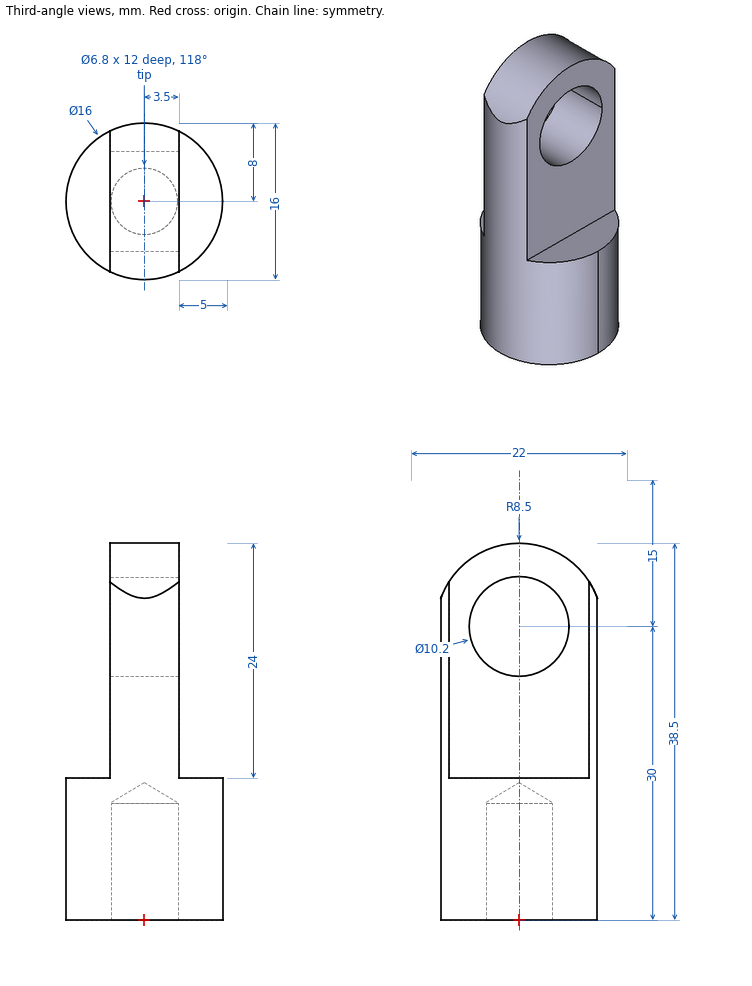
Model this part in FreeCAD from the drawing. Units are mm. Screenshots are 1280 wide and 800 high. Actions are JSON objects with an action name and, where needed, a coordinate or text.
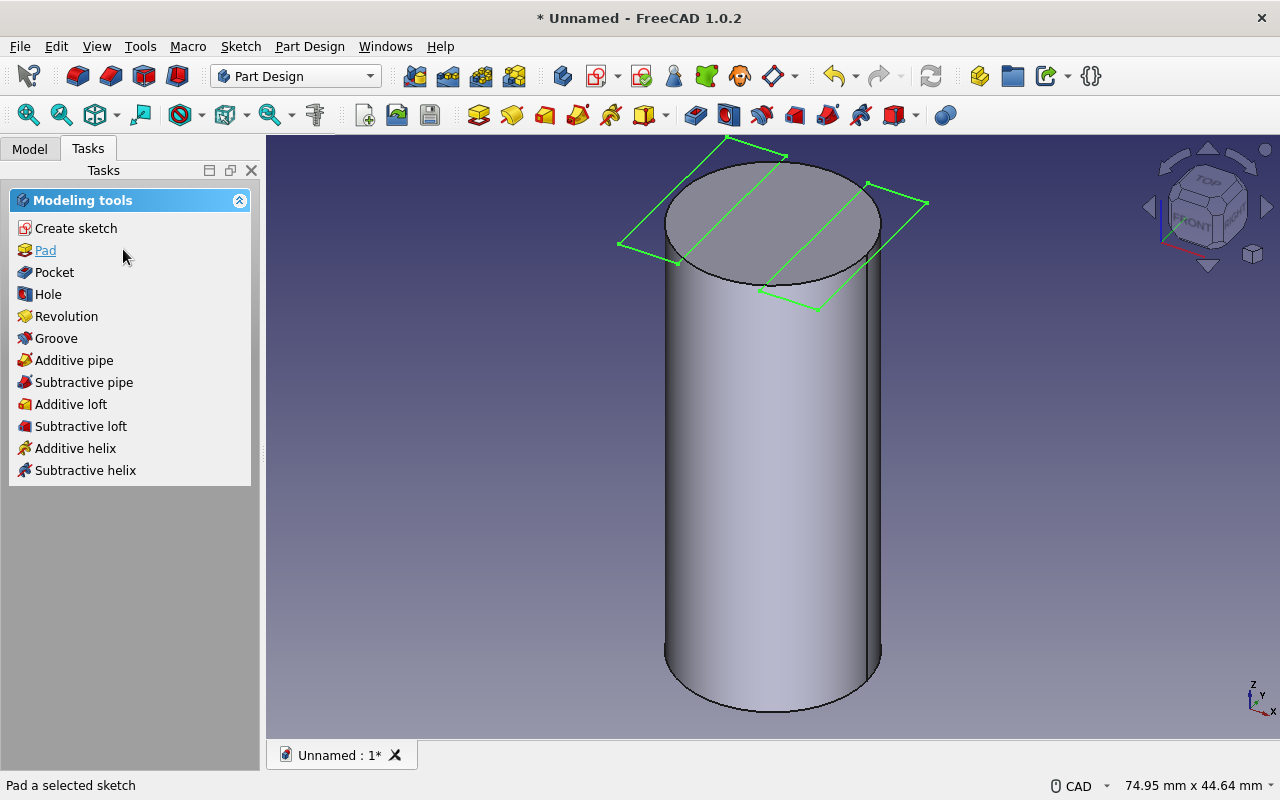
{"action": "left_click", "coordinate": [696, 116]}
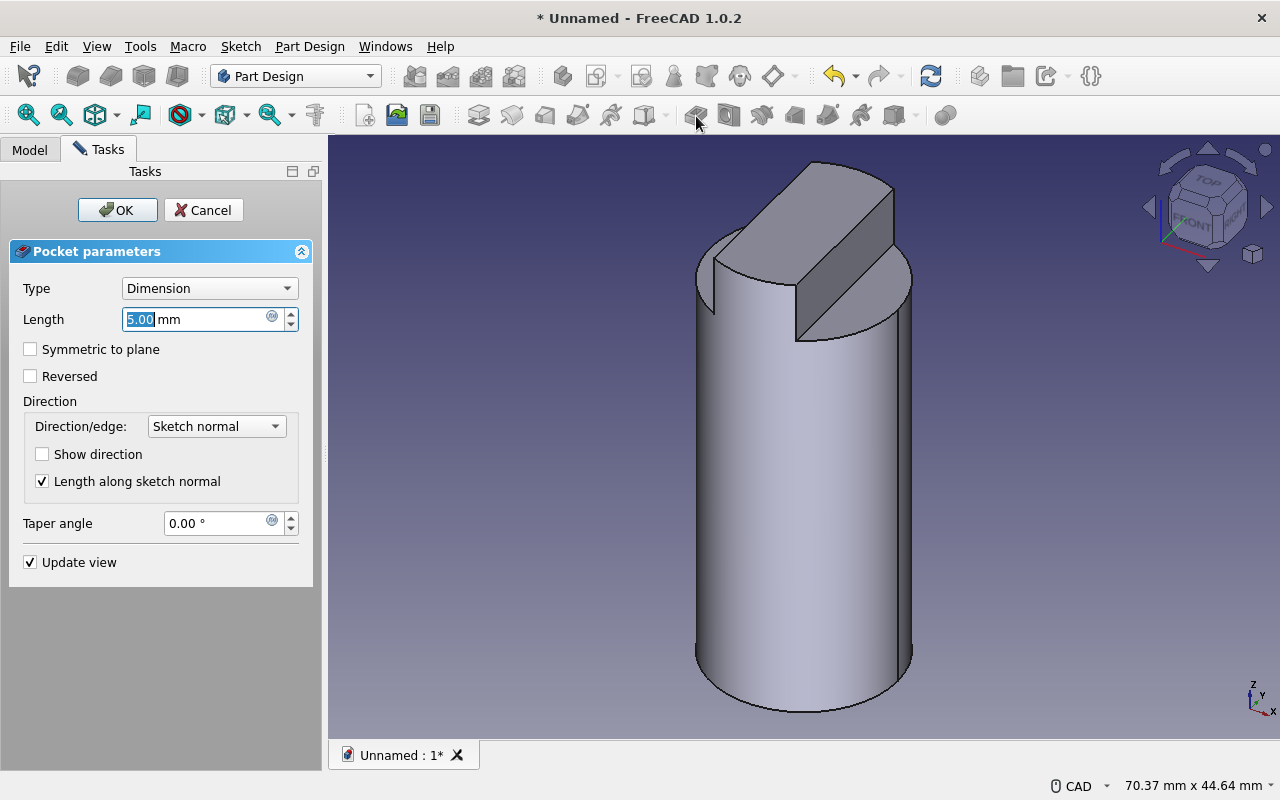
{"action": "type", "text": "24"}
{"action": "key", "text": "Tab"}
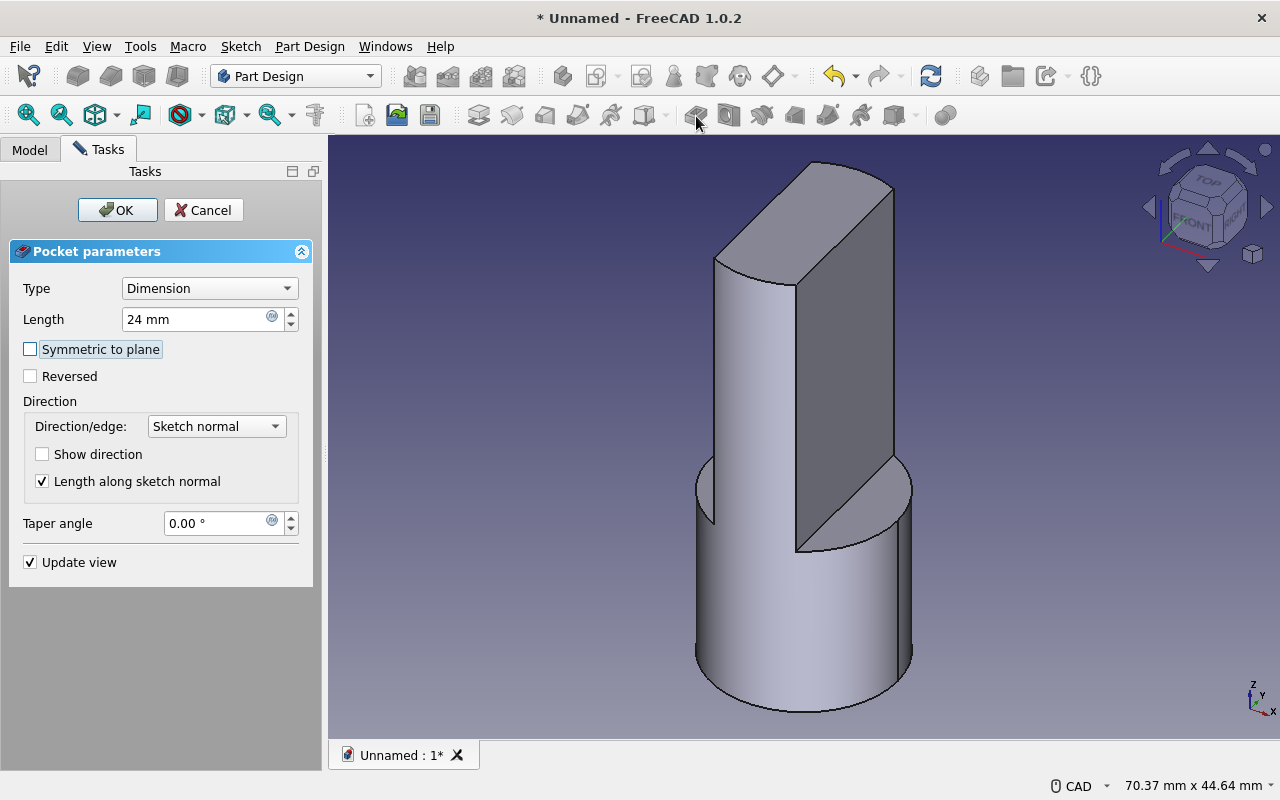
{"action": "left_click", "coordinate": [118, 210]}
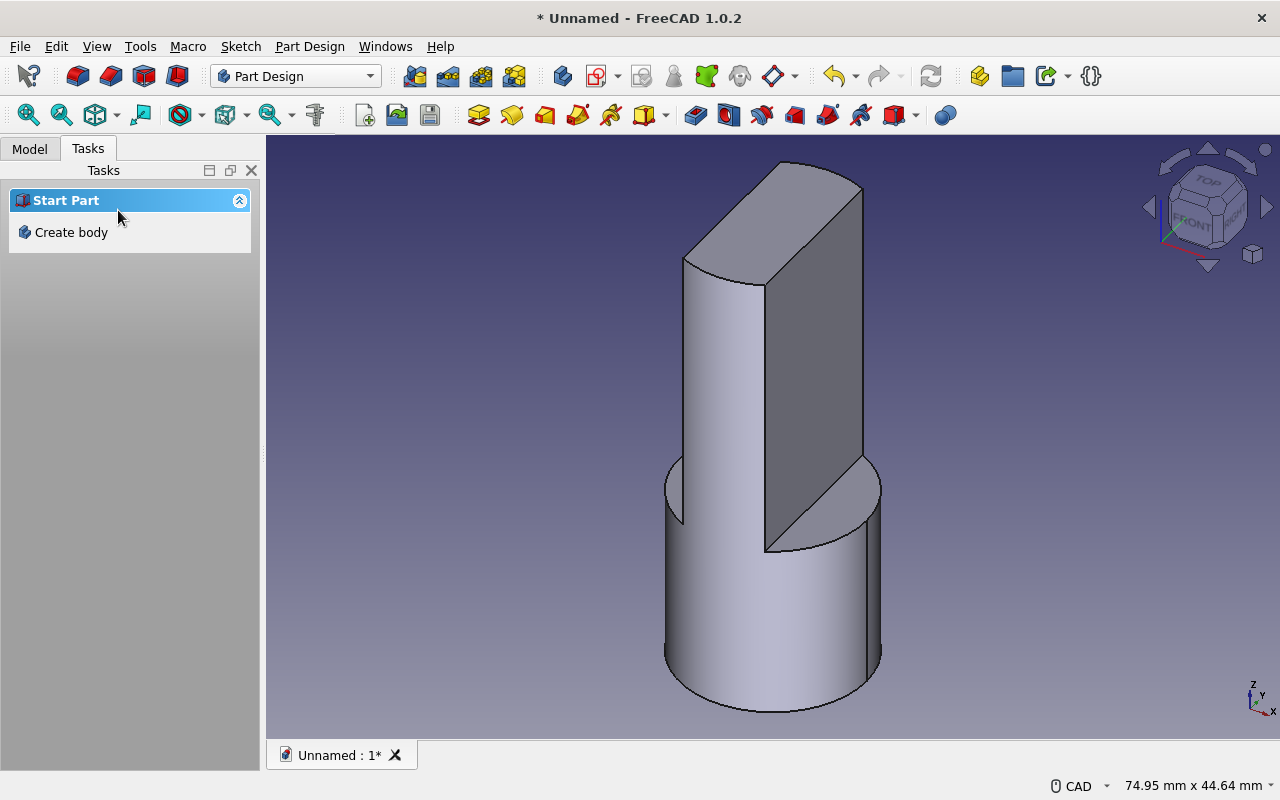
{"action": "left_click", "coordinate": [814, 331]}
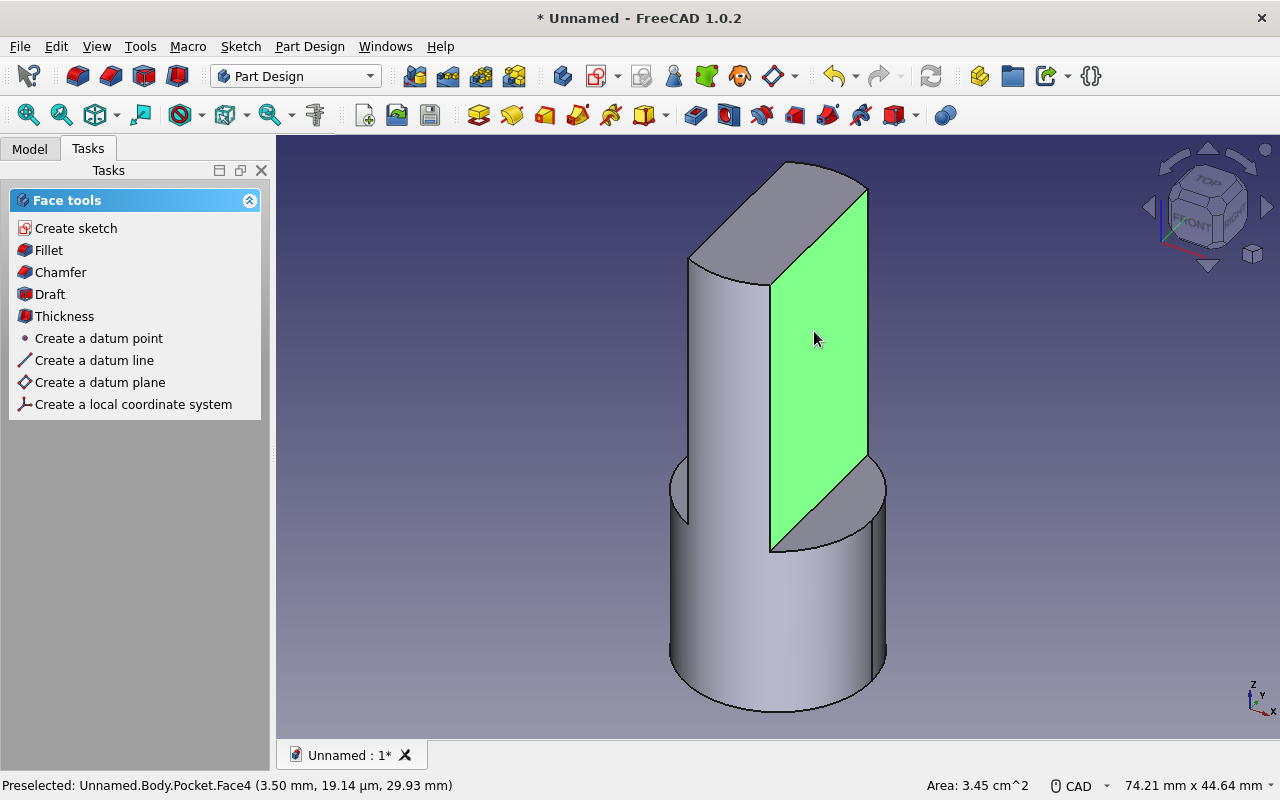
{"action": "left_click", "coordinate": [596, 76]}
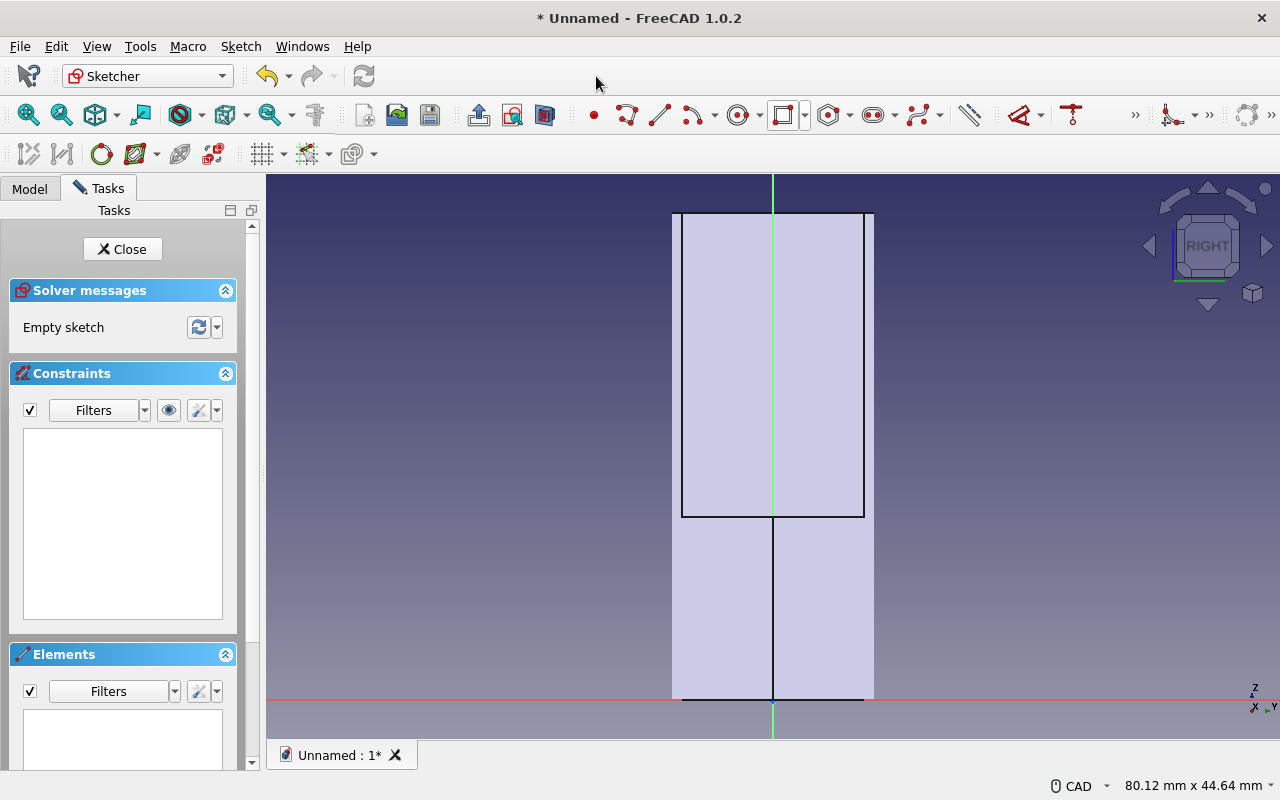
{"action": "scroll", "coordinate": [813, 241], "scroll_direction": "up", "scroll_amount": 5}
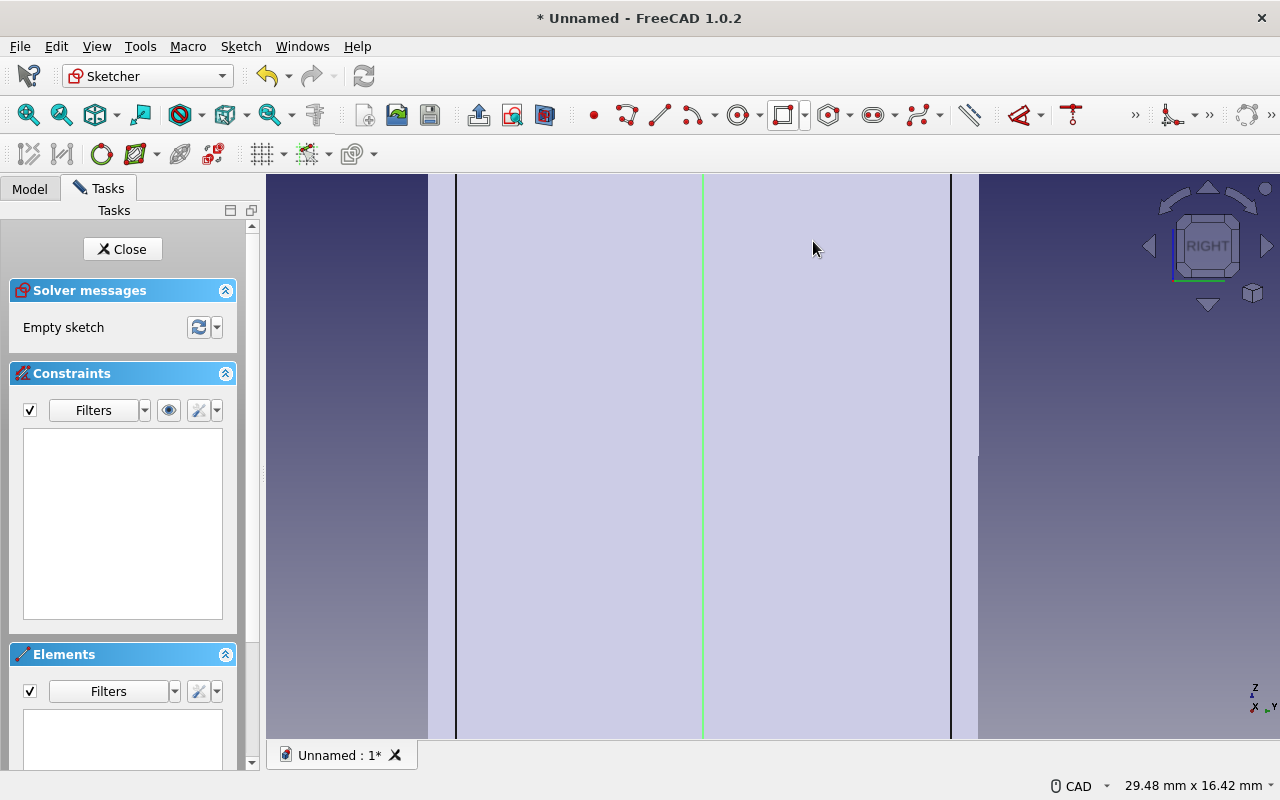
{"action": "key", "text": "g c"}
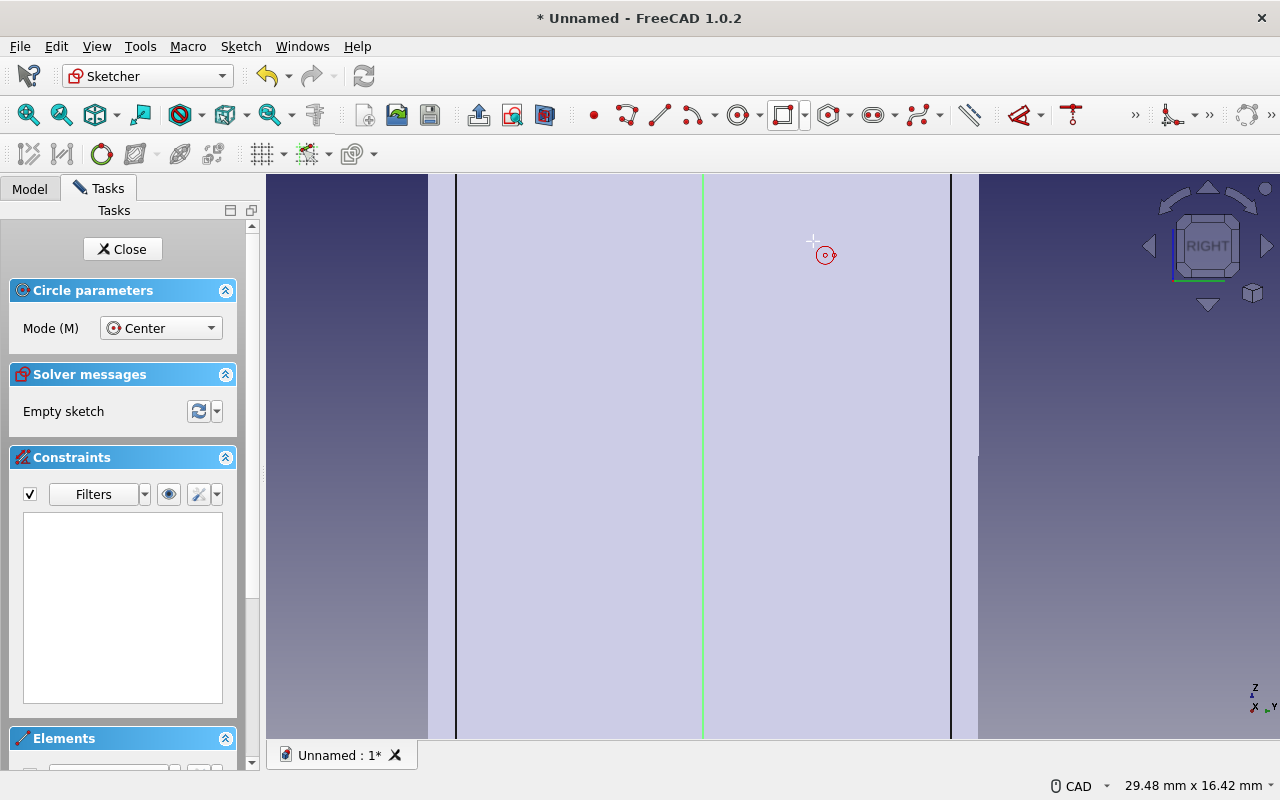
{"action": "left_click", "coordinate": [703, 457]}
{"action": "left_click", "coordinate": [827, 333]}
{"action": "key", "text": "Escape"}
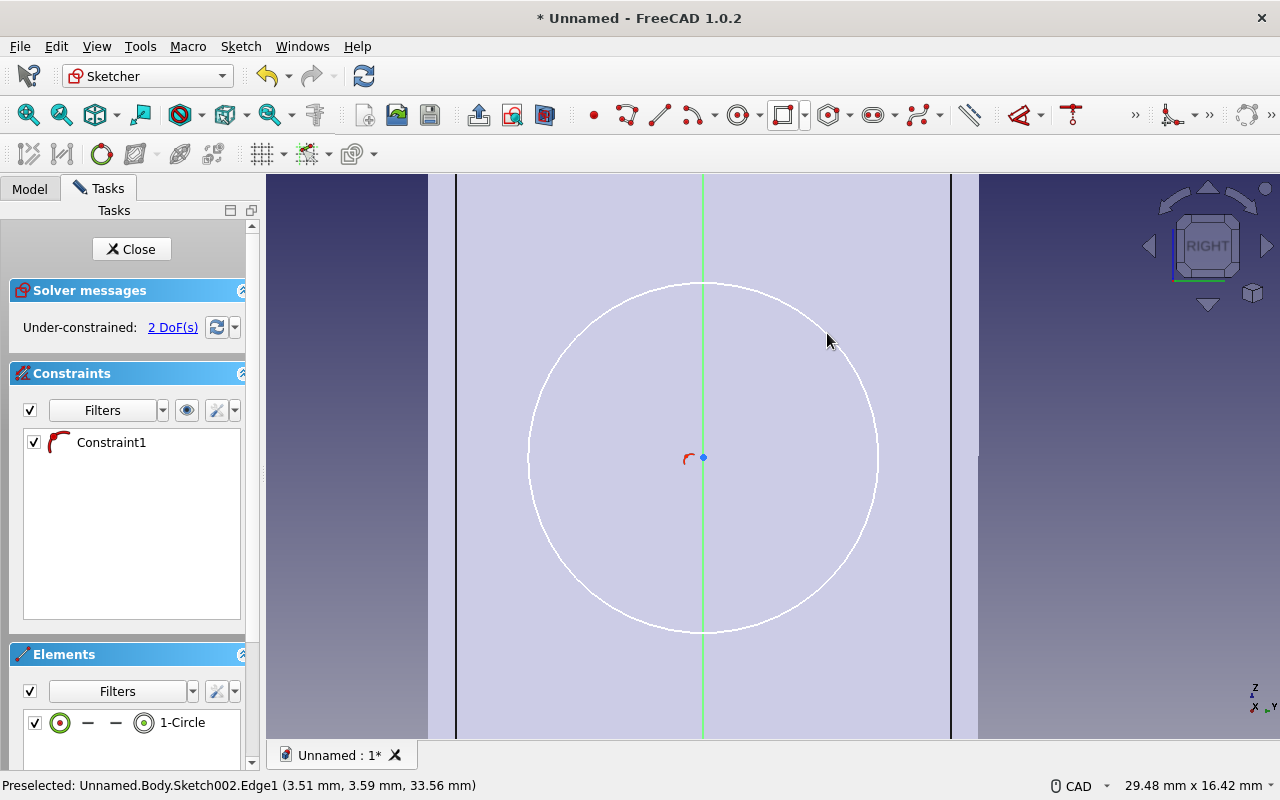
{"action": "key", "text": "d"}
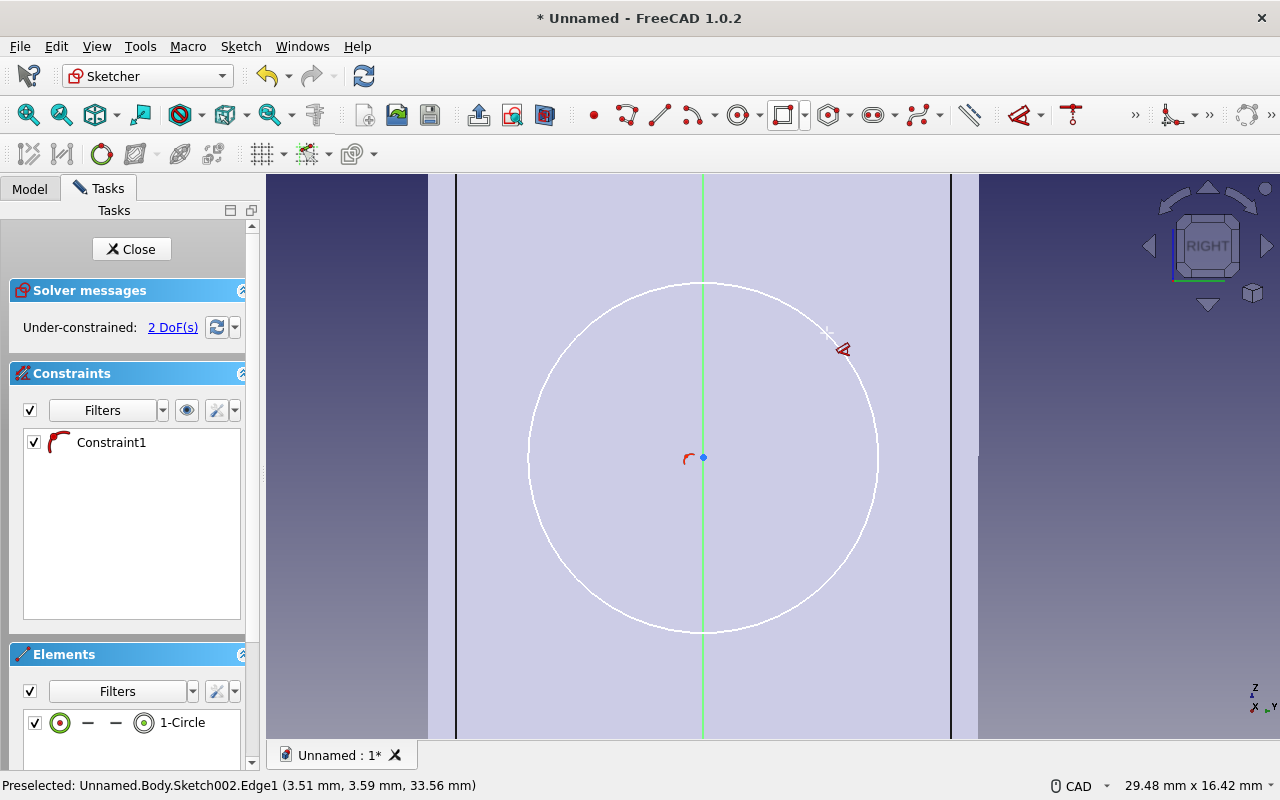
{"action": "left_click", "coordinate": [827, 334]}
{"action": "left_click", "coordinate": [850, 311]}